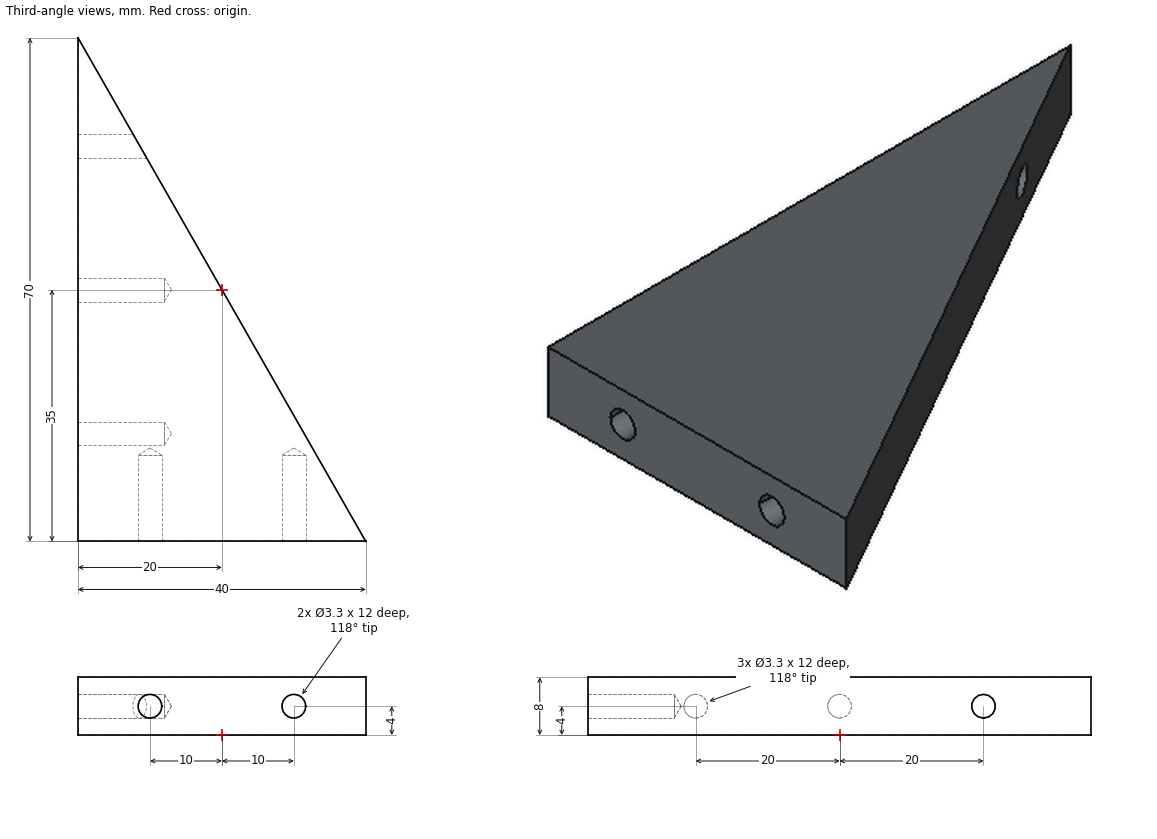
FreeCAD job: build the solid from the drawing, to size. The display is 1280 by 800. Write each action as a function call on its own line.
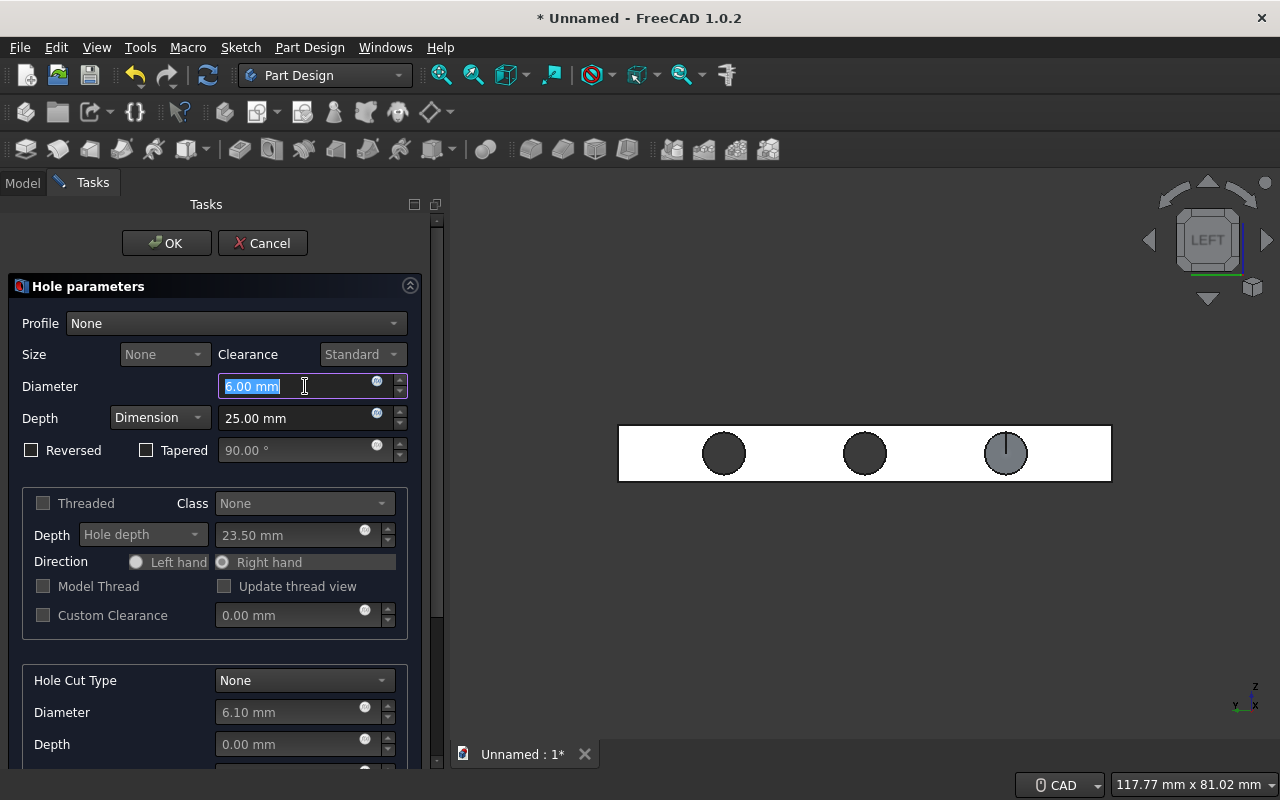
text(3.3)
key(Tab)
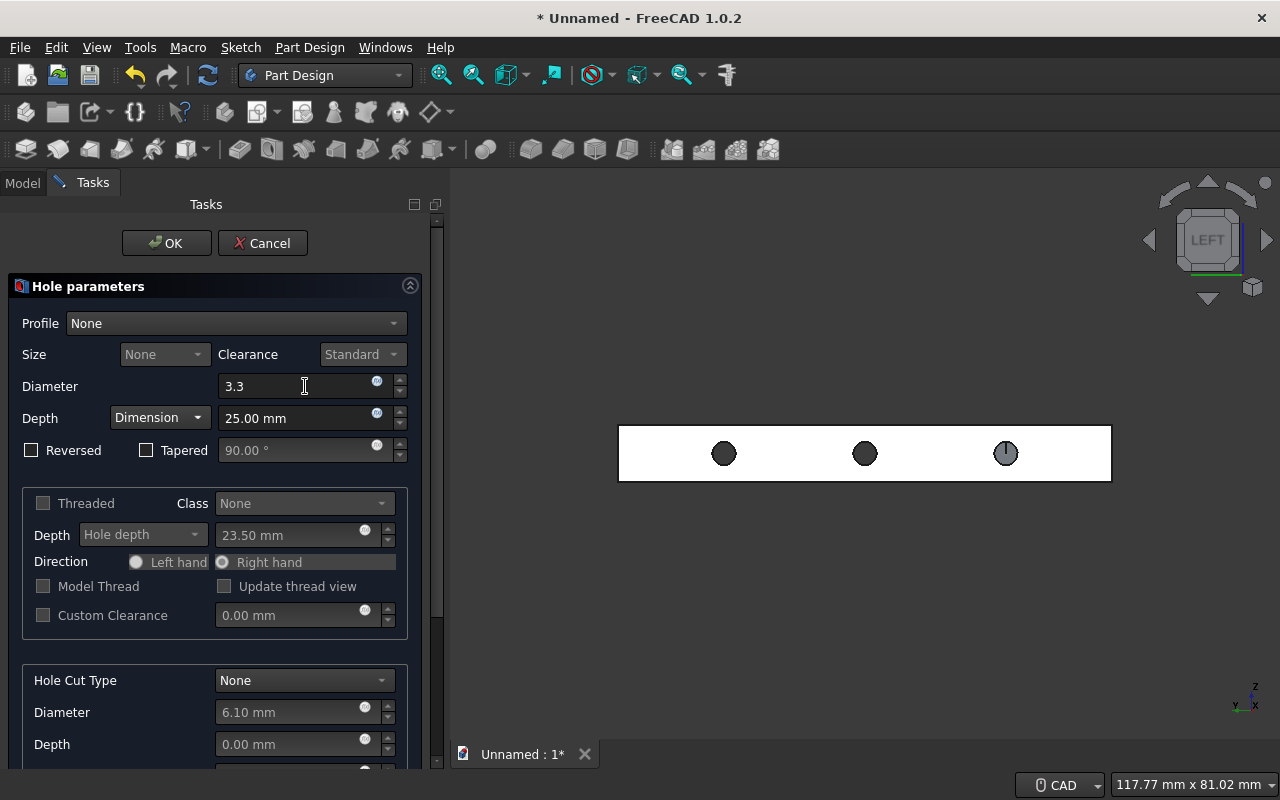
triple_click(305, 418)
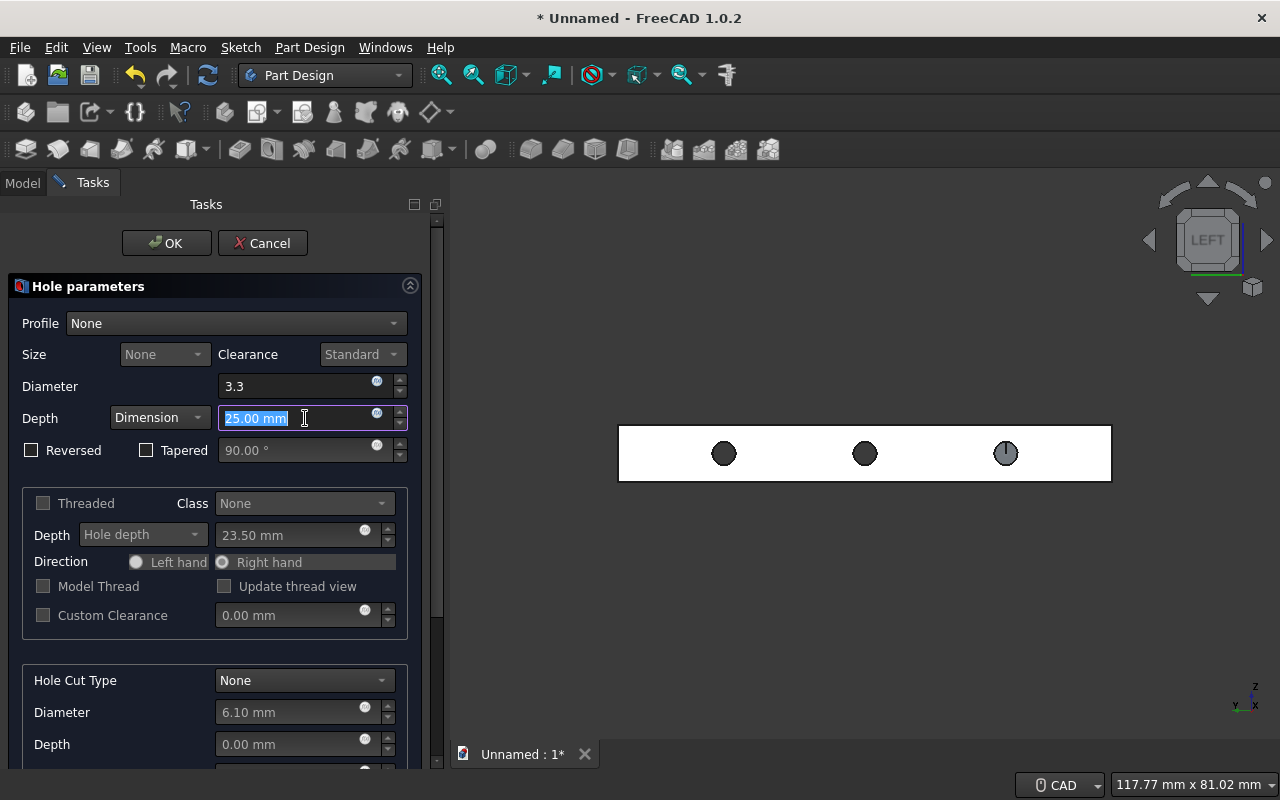
text(12)
key(Tab)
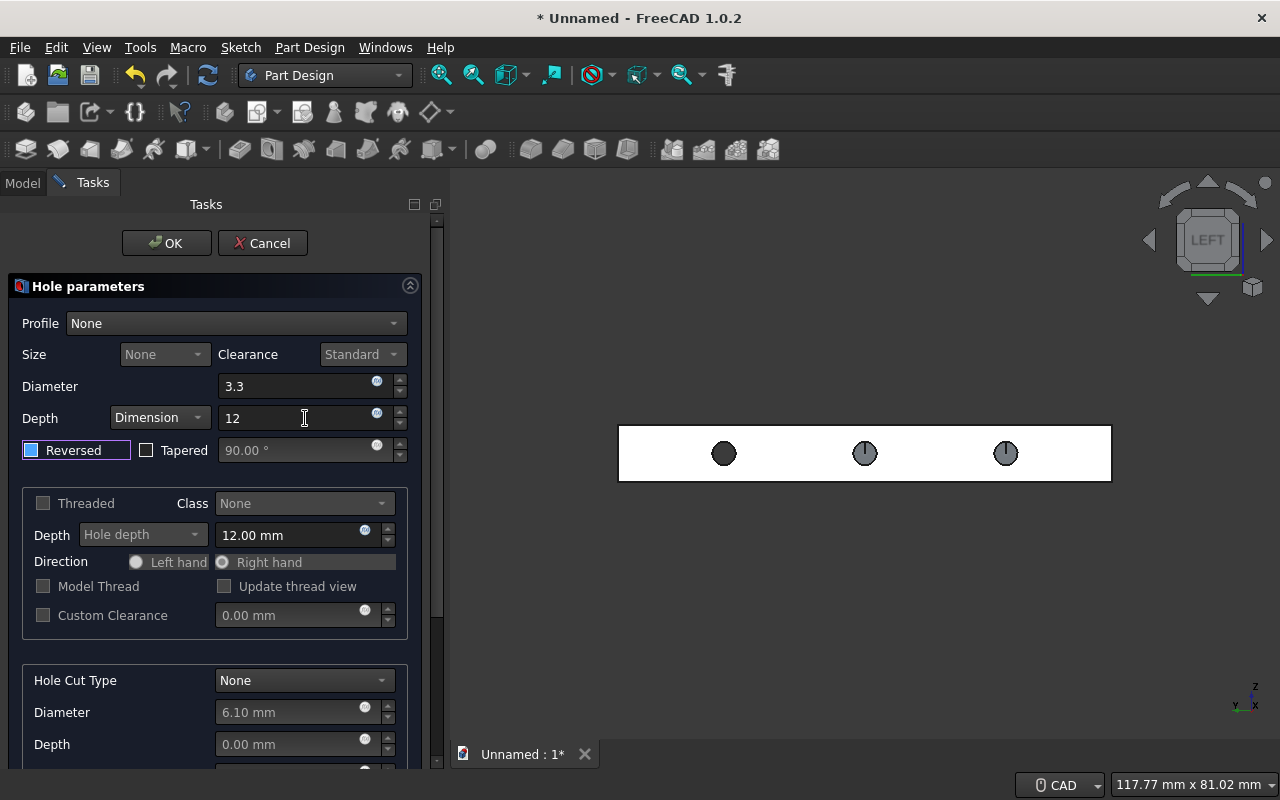
click(167, 243)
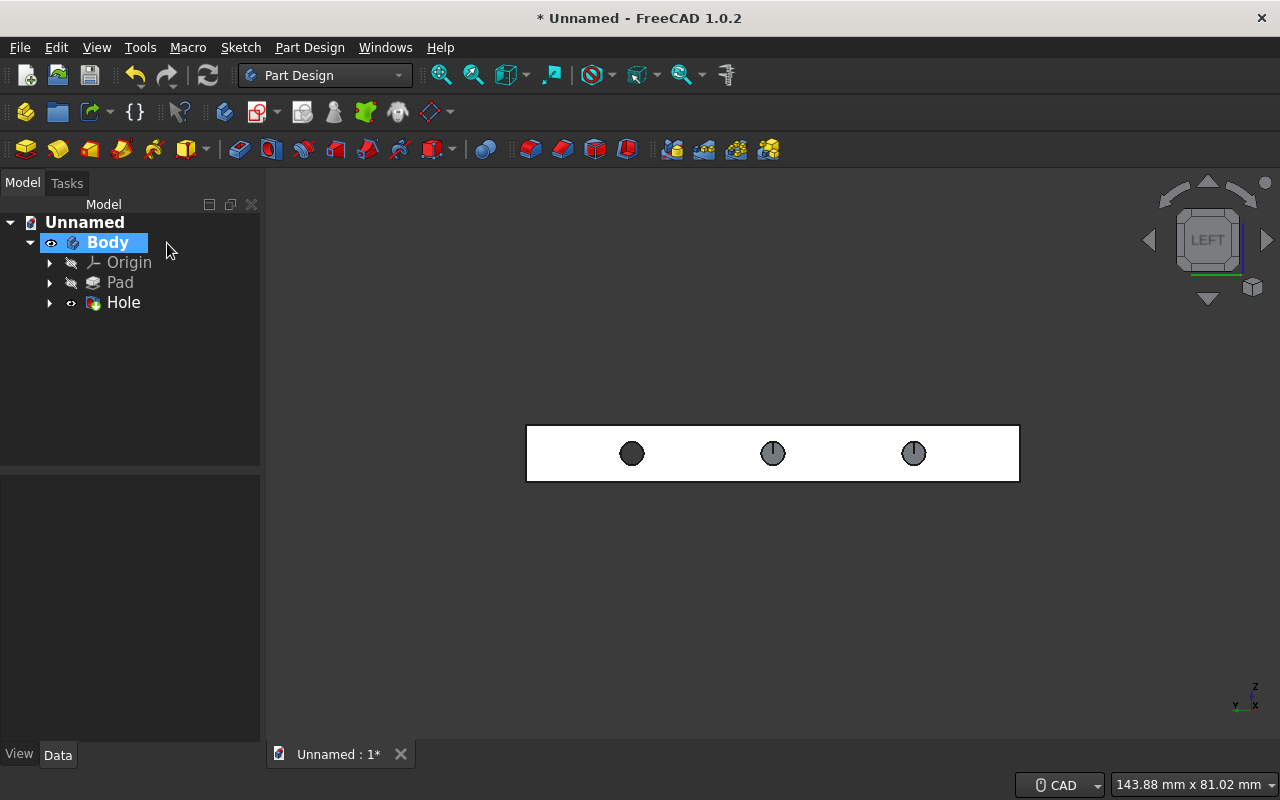
key(0)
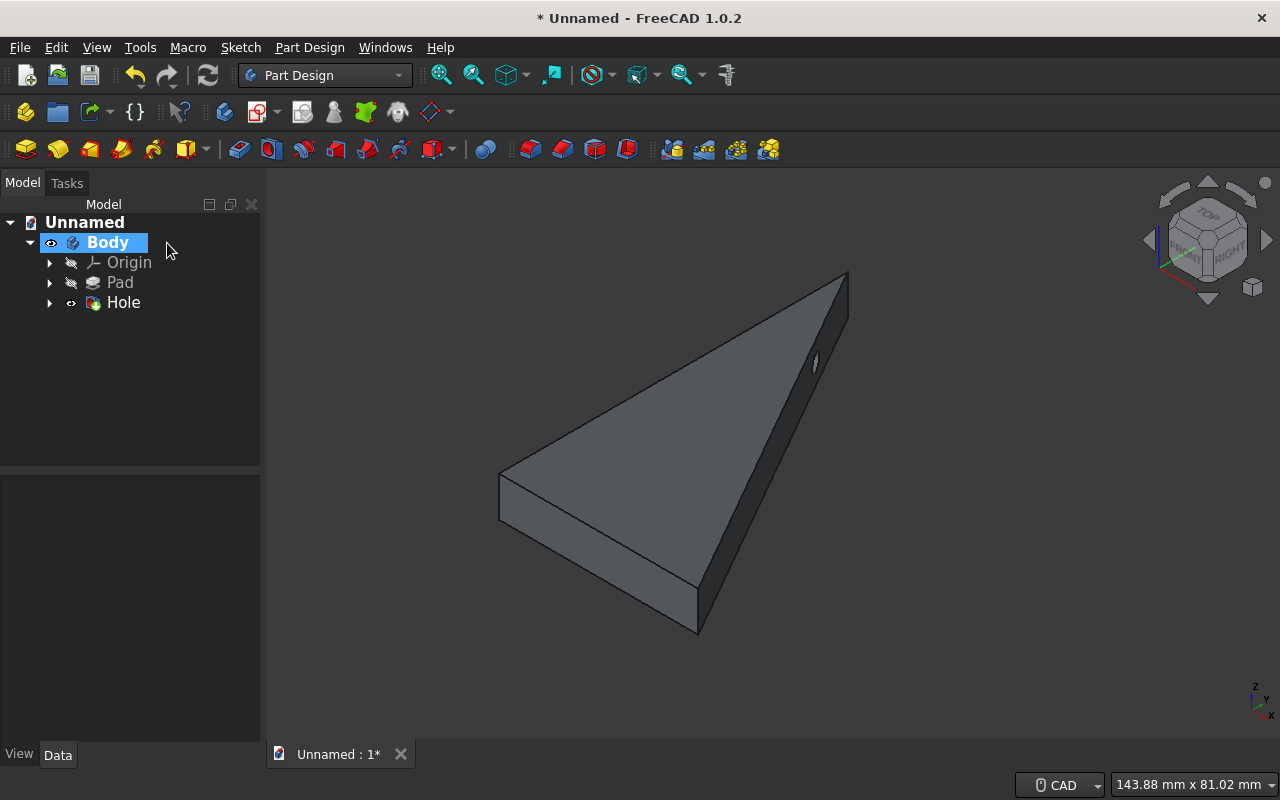
click(656, 586)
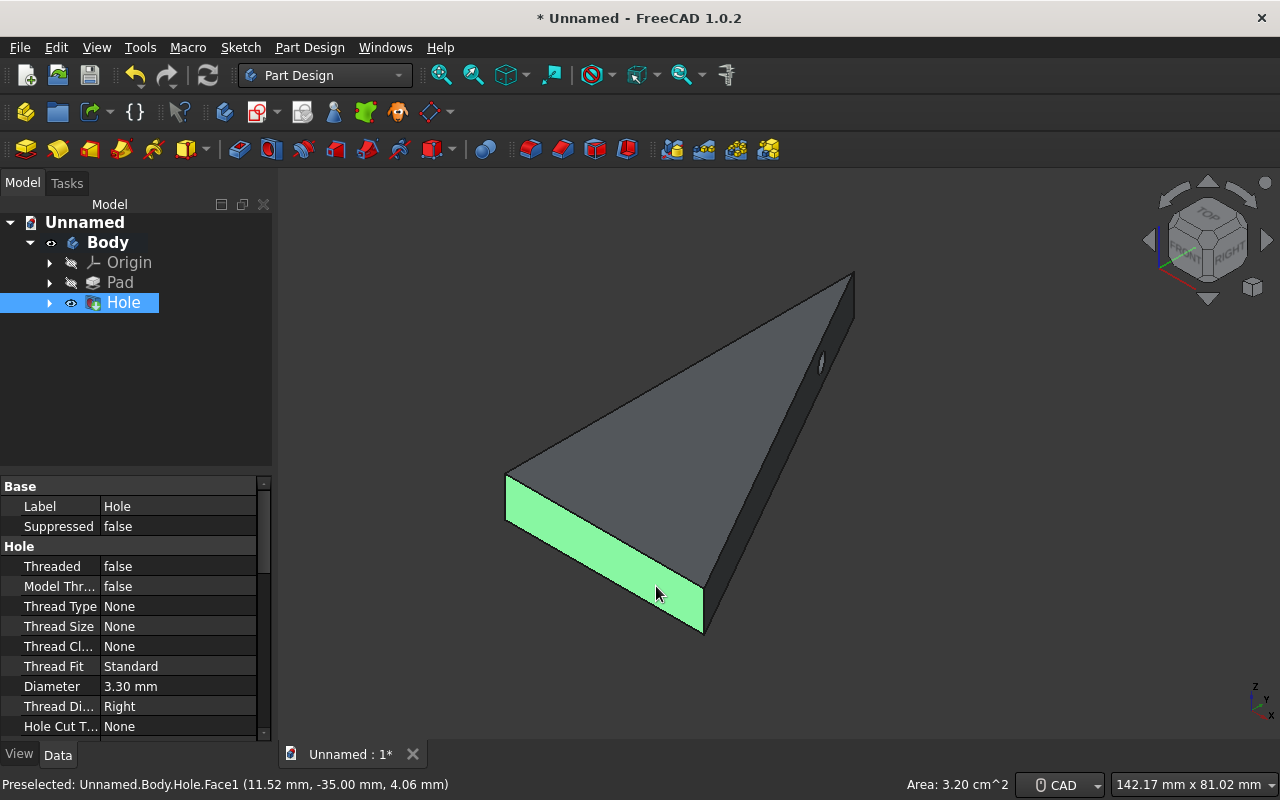
click(258, 112)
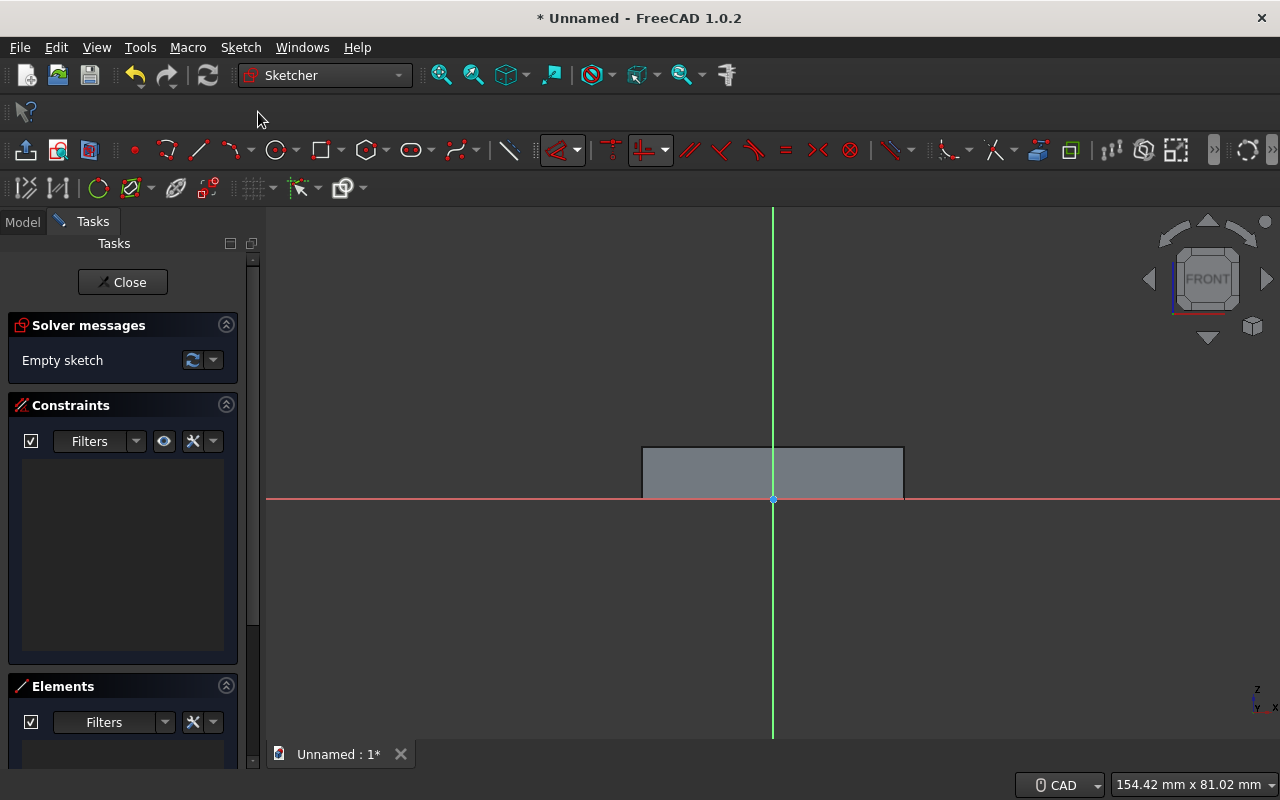
scroll(795, 483, up, 7)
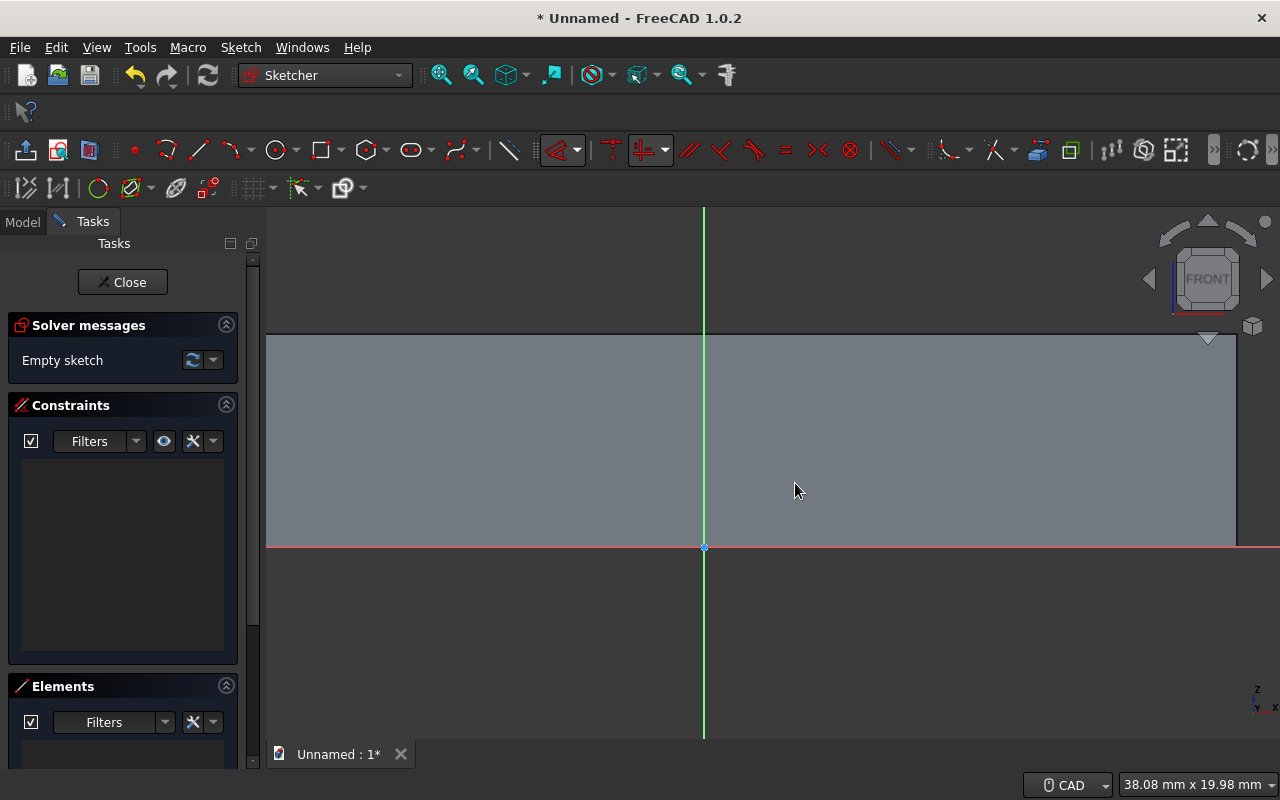
click(276, 150)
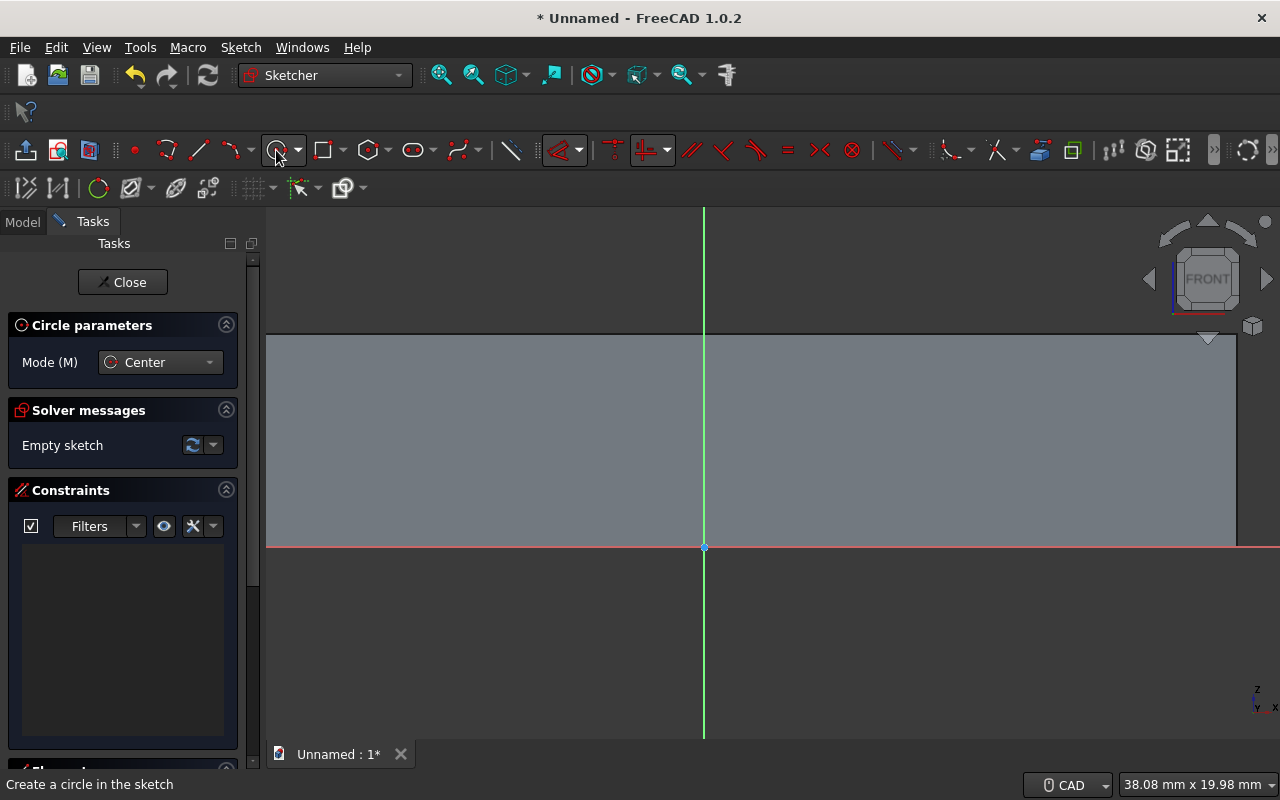
click(970, 441)
click(1002, 410)